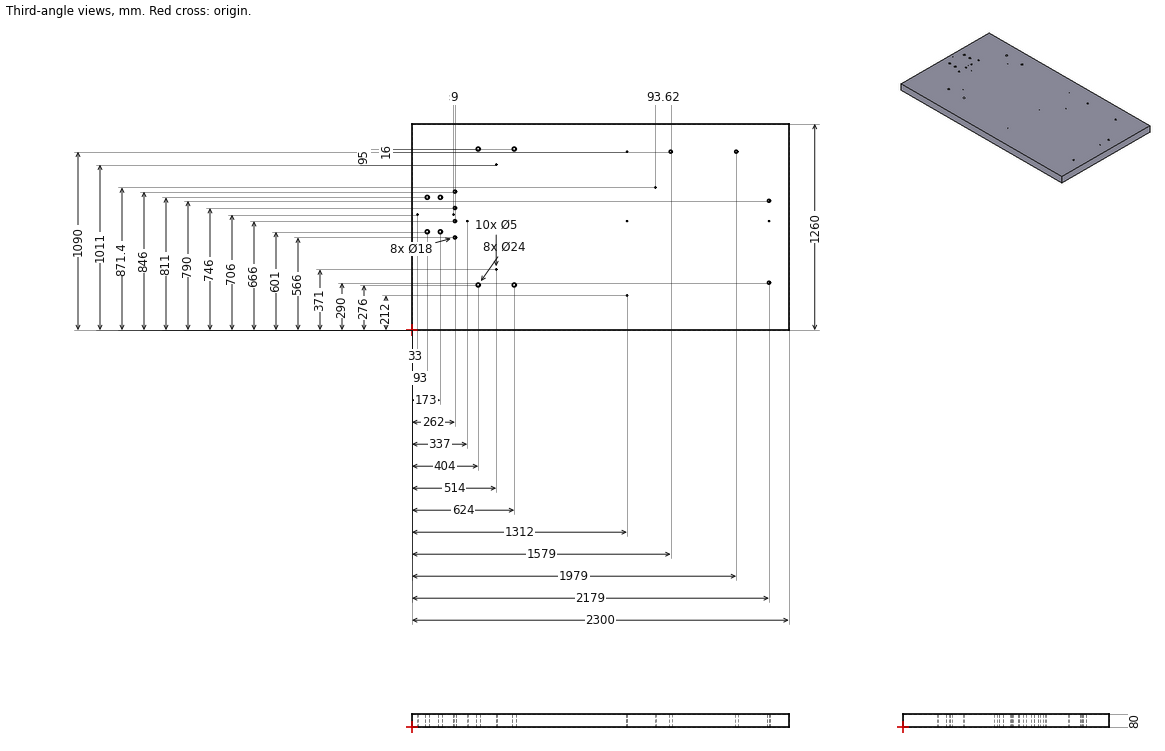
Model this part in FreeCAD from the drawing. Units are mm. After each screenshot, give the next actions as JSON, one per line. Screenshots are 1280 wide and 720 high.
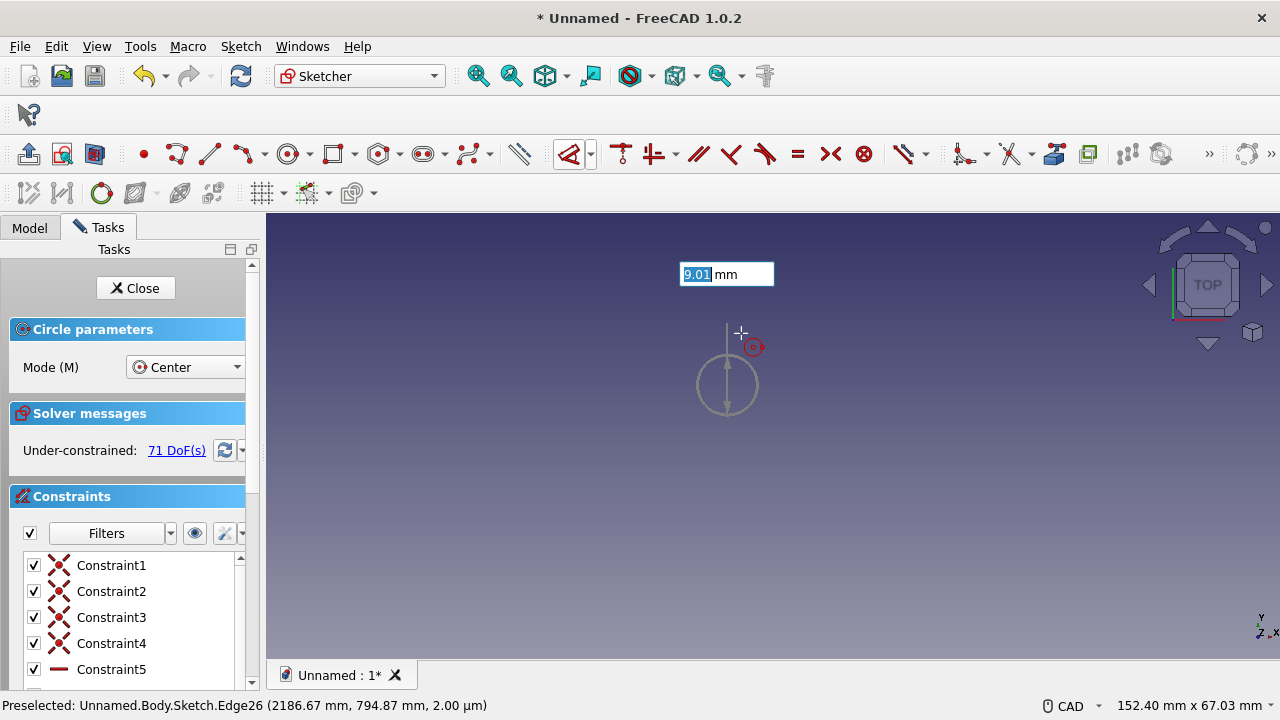
{"action": "left_click", "coordinate": [732, 337]}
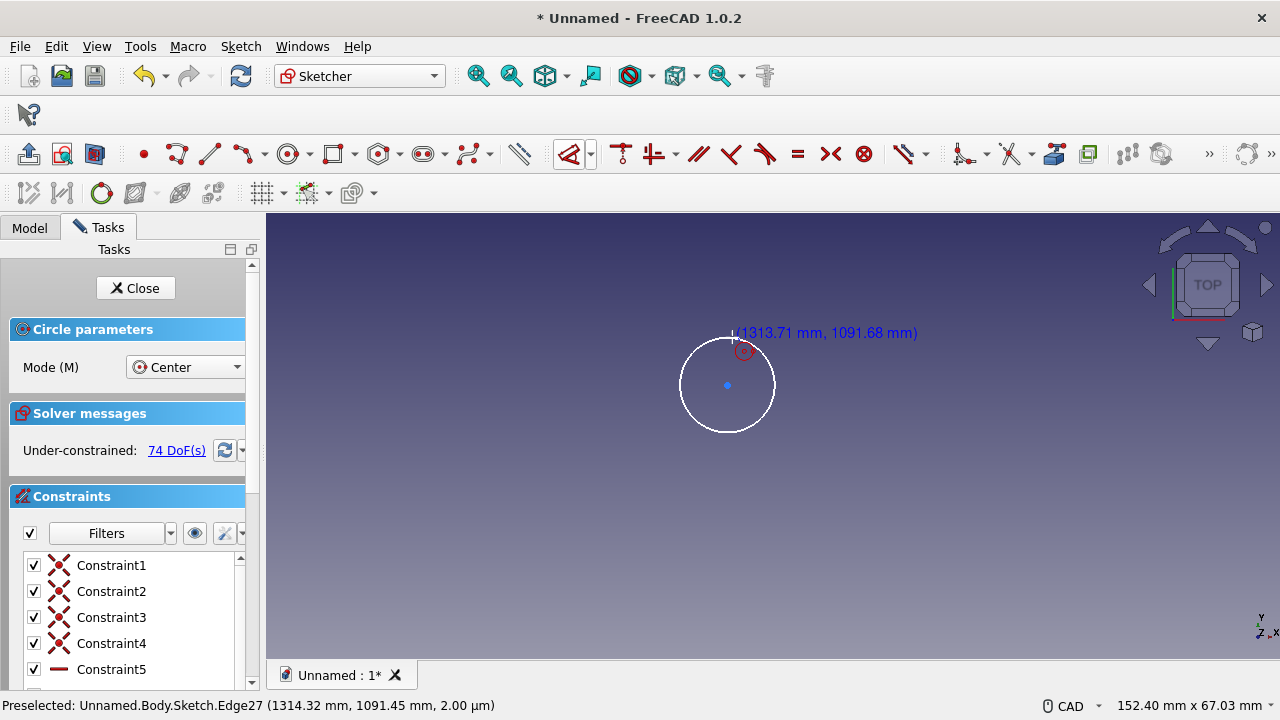
{"action": "scroll", "coordinate": [741, 333], "scroll_direction": "down", "scroll_amount": 17}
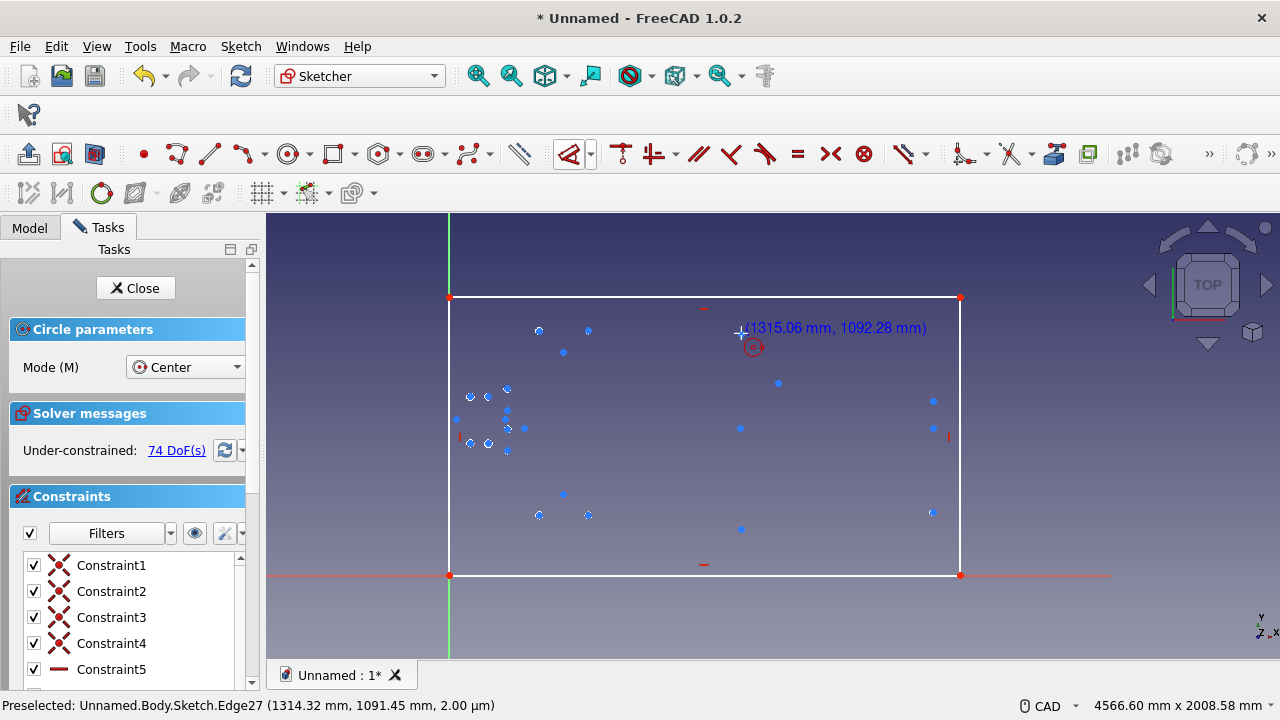
{"action": "scroll", "coordinate": [800, 334], "scroll_direction": "up", "scroll_amount": 13}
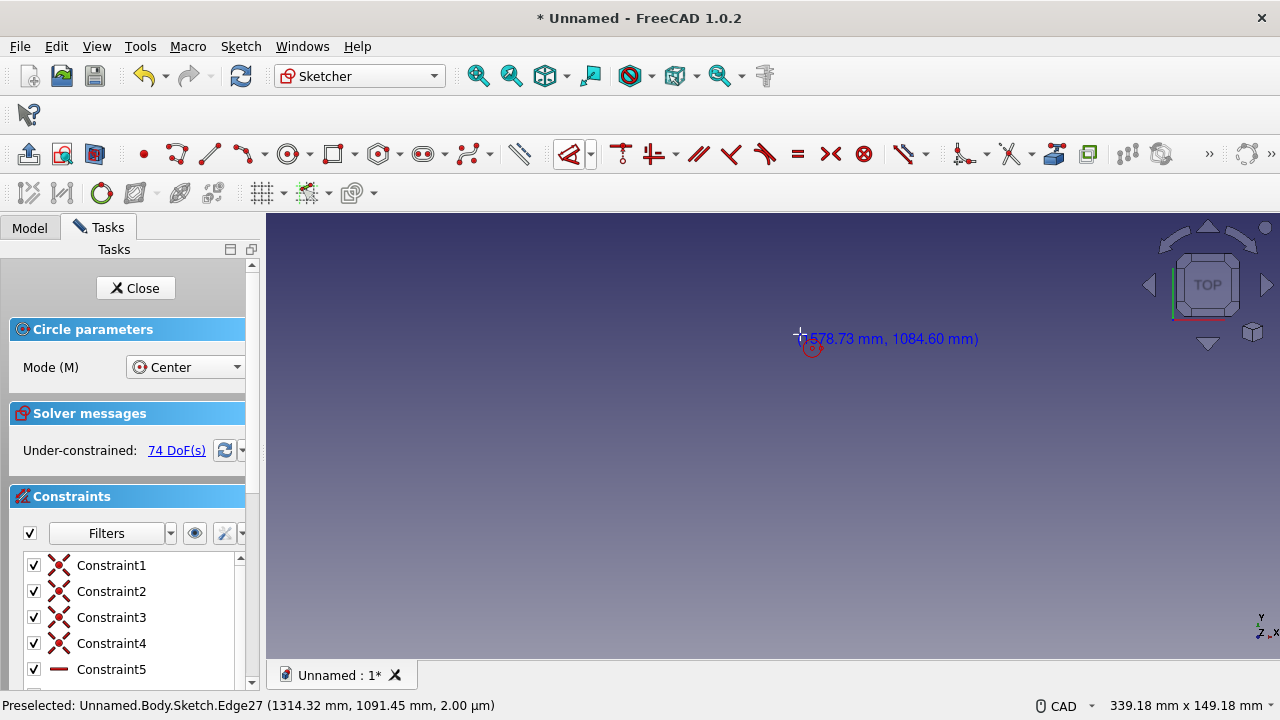
{"action": "scroll", "coordinate": [800, 334], "scroll_direction": "down", "scroll_amount": 13}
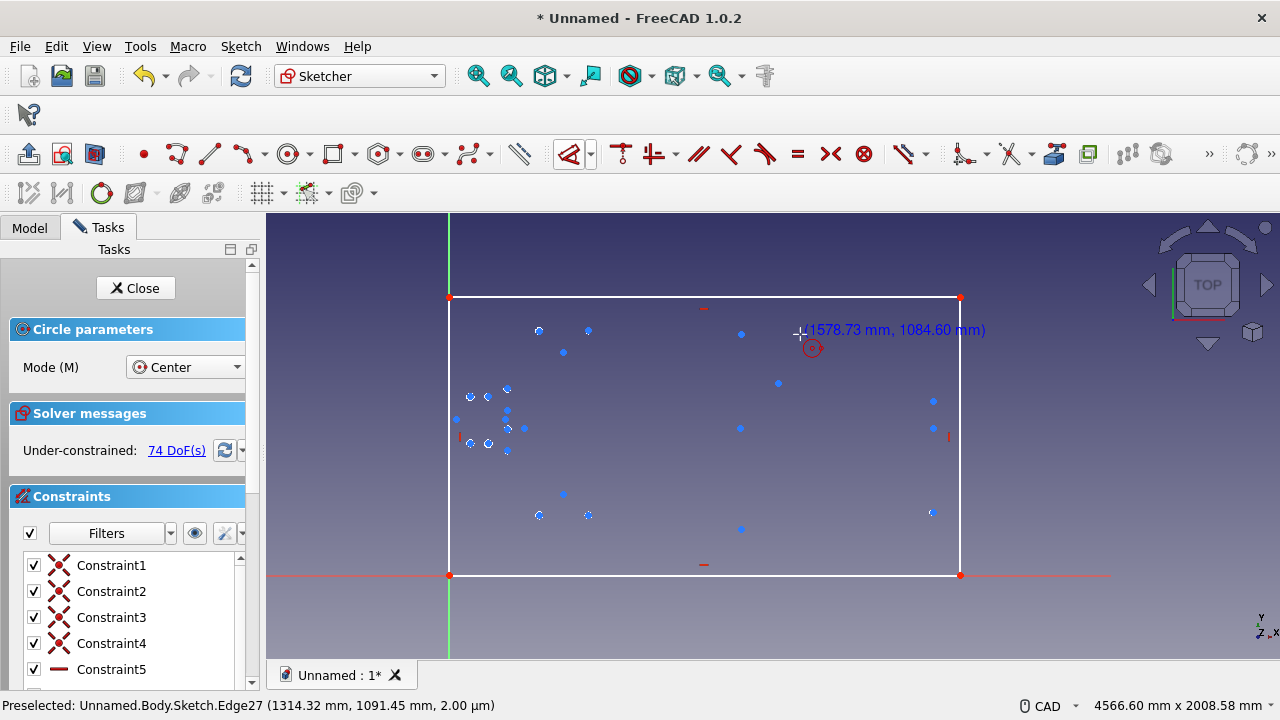
{"action": "left_click", "coordinate": [800, 334]}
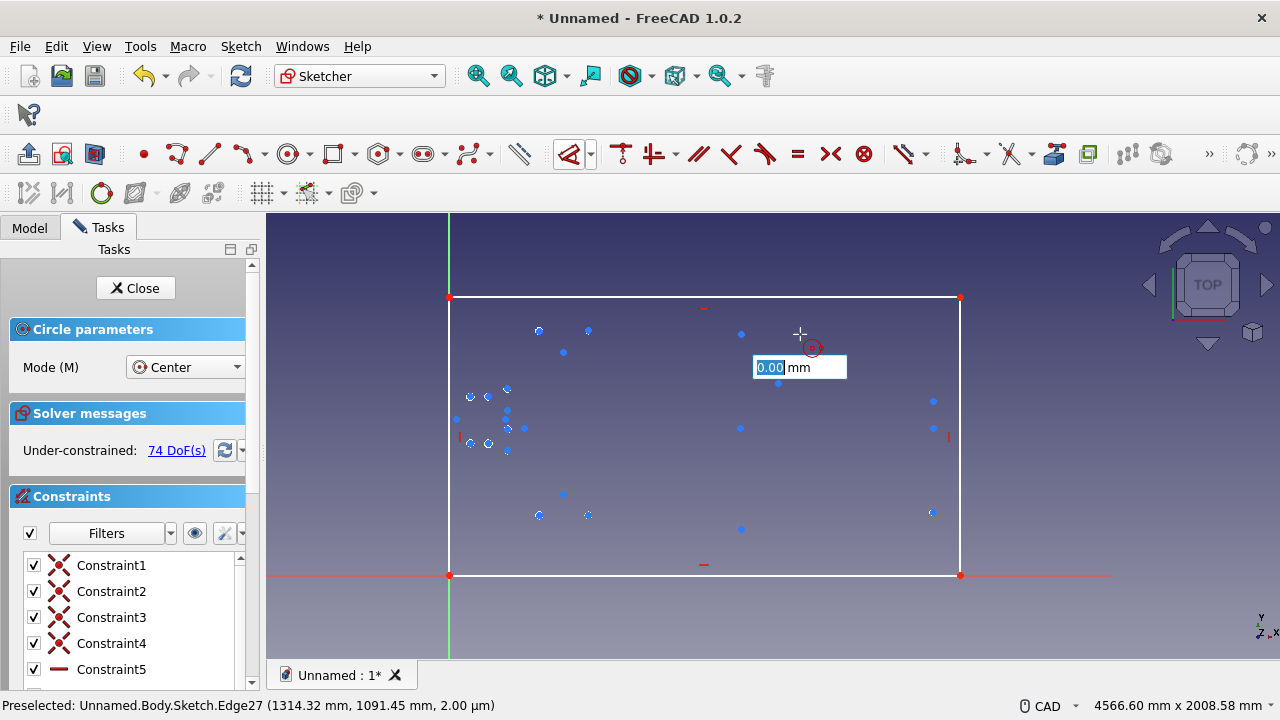
{"action": "scroll", "coordinate": [801, 332], "scroll_direction": "up", "scroll_amount": 11}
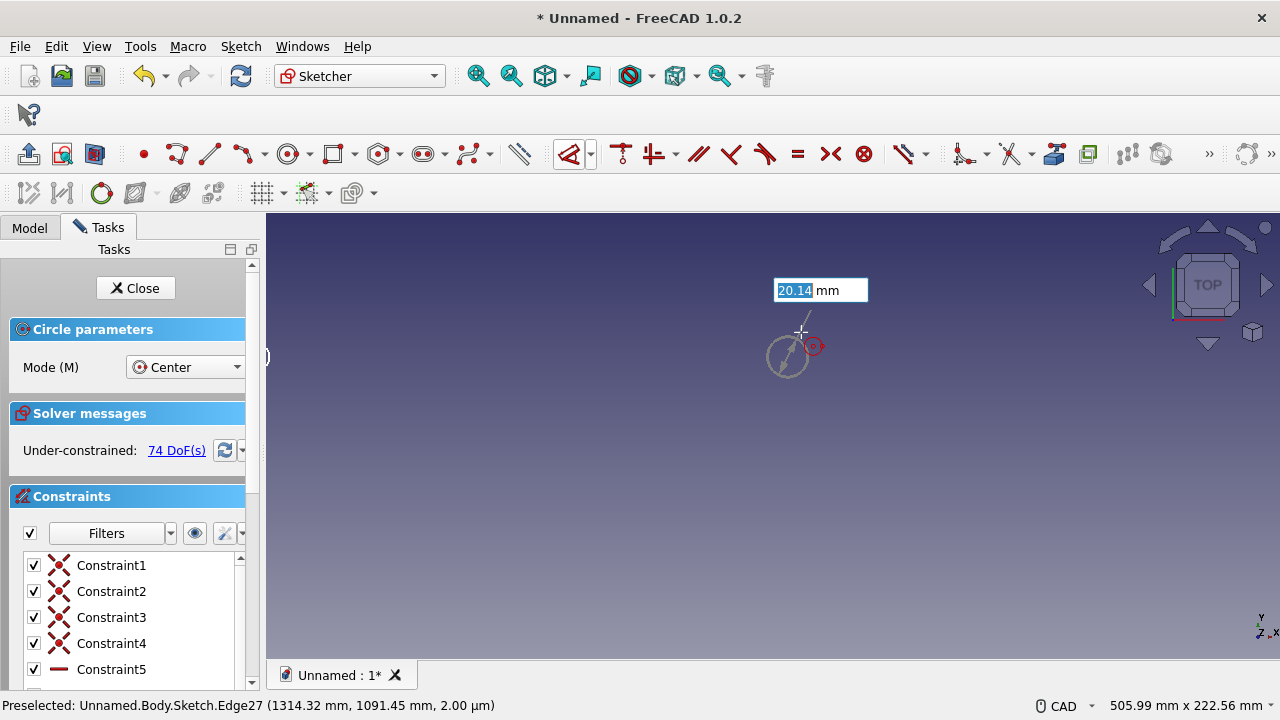
{"action": "left_click", "coordinate": [801, 333]}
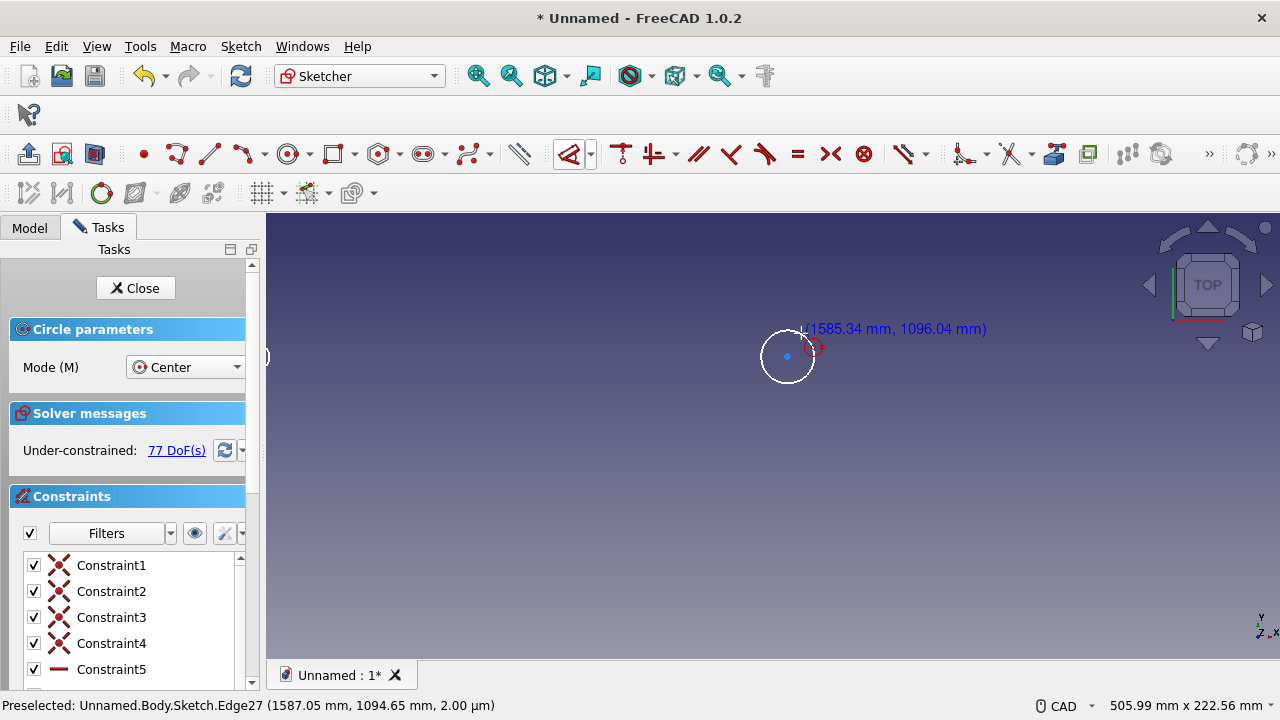
{"action": "scroll", "coordinate": [801, 332], "scroll_direction": "down", "scroll_amount": 11}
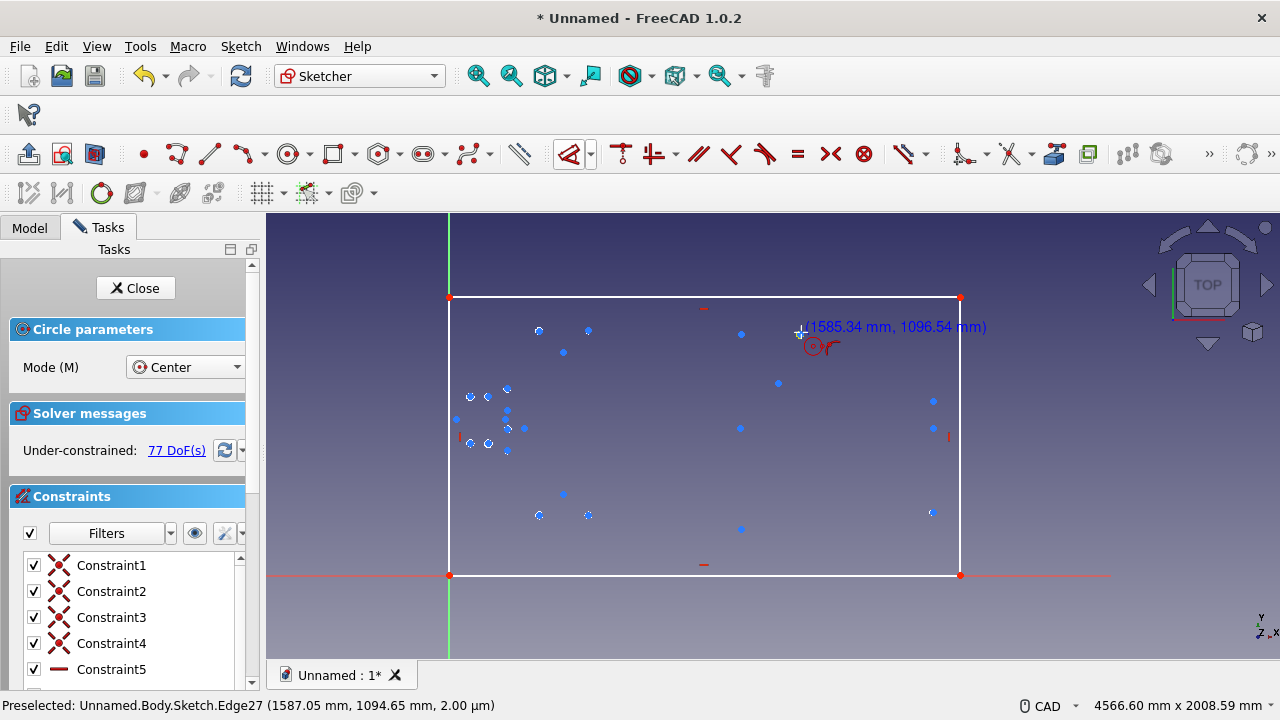
{"action": "scroll", "coordinate": [889, 334], "scroll_direction": "up", "scroll_amount": 13}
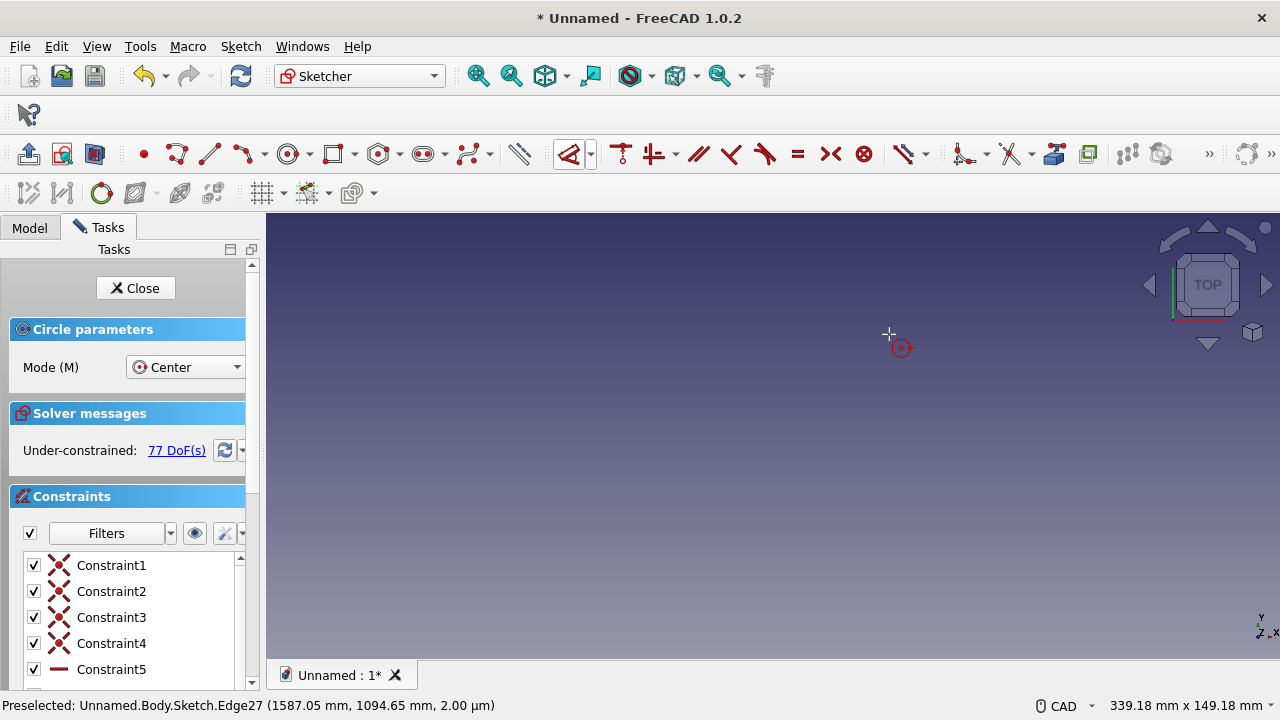
{"action": "scroll", "coordinate": [889, 334], "scroll_direction": "down", "scroll_amount": 13}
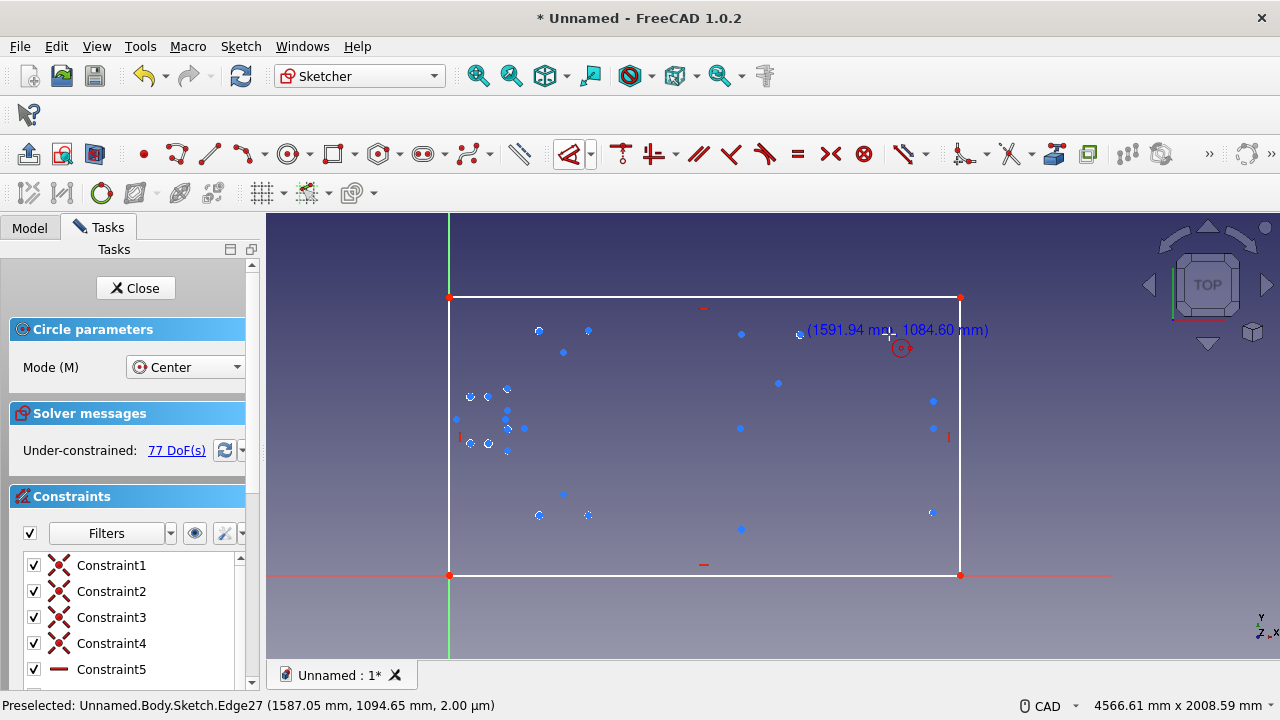
{"action": "left_click", "coordinate": [889, 334]}